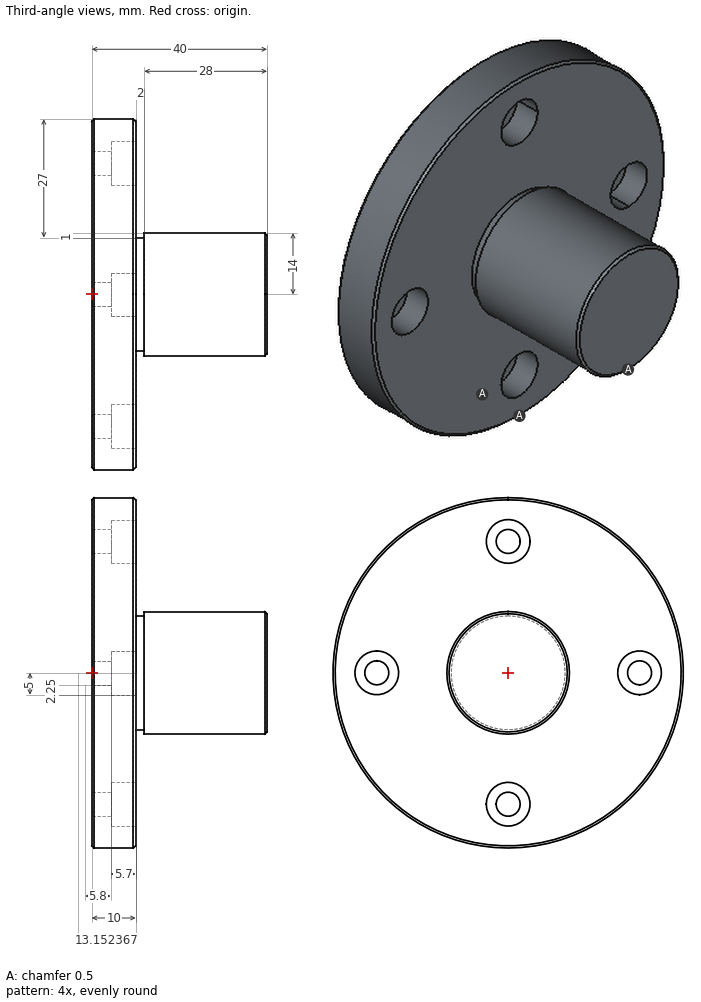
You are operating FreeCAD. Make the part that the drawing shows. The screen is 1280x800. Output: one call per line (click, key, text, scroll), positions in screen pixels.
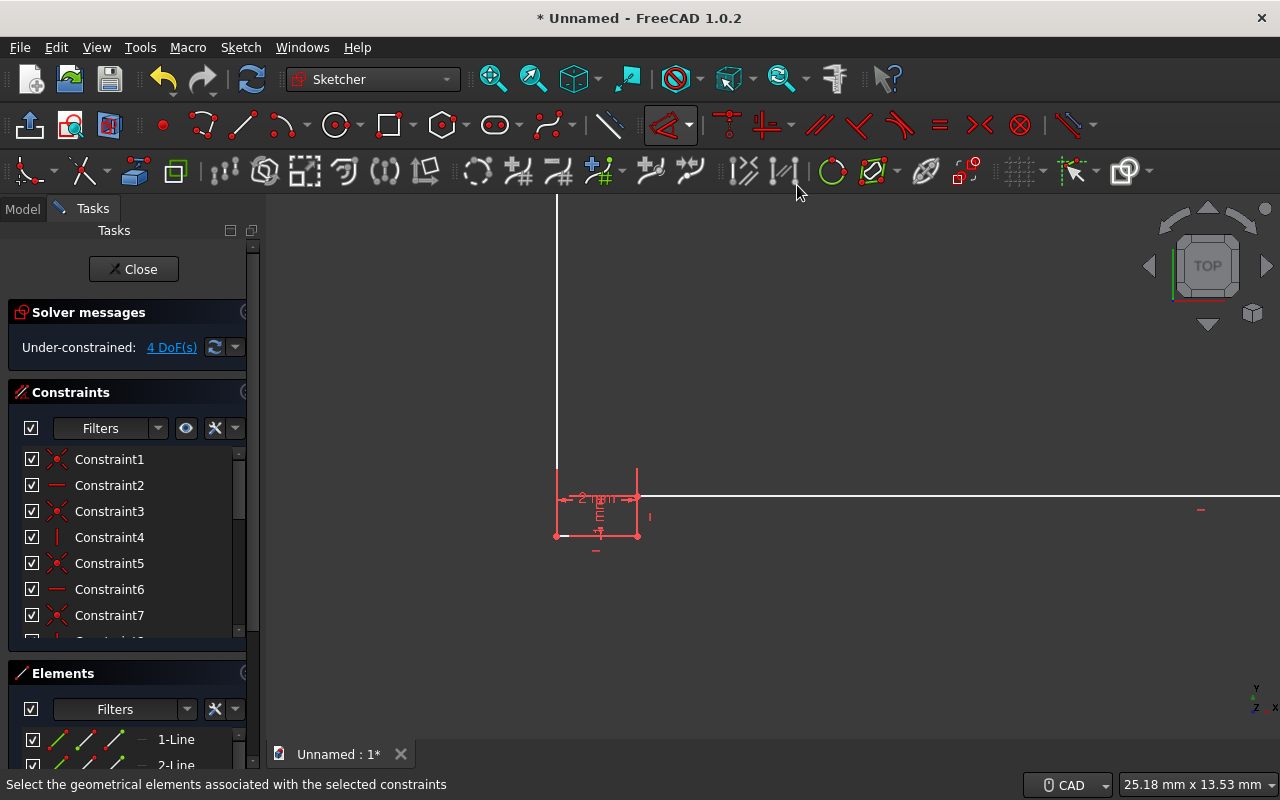
scroll(640, 520, down, 8)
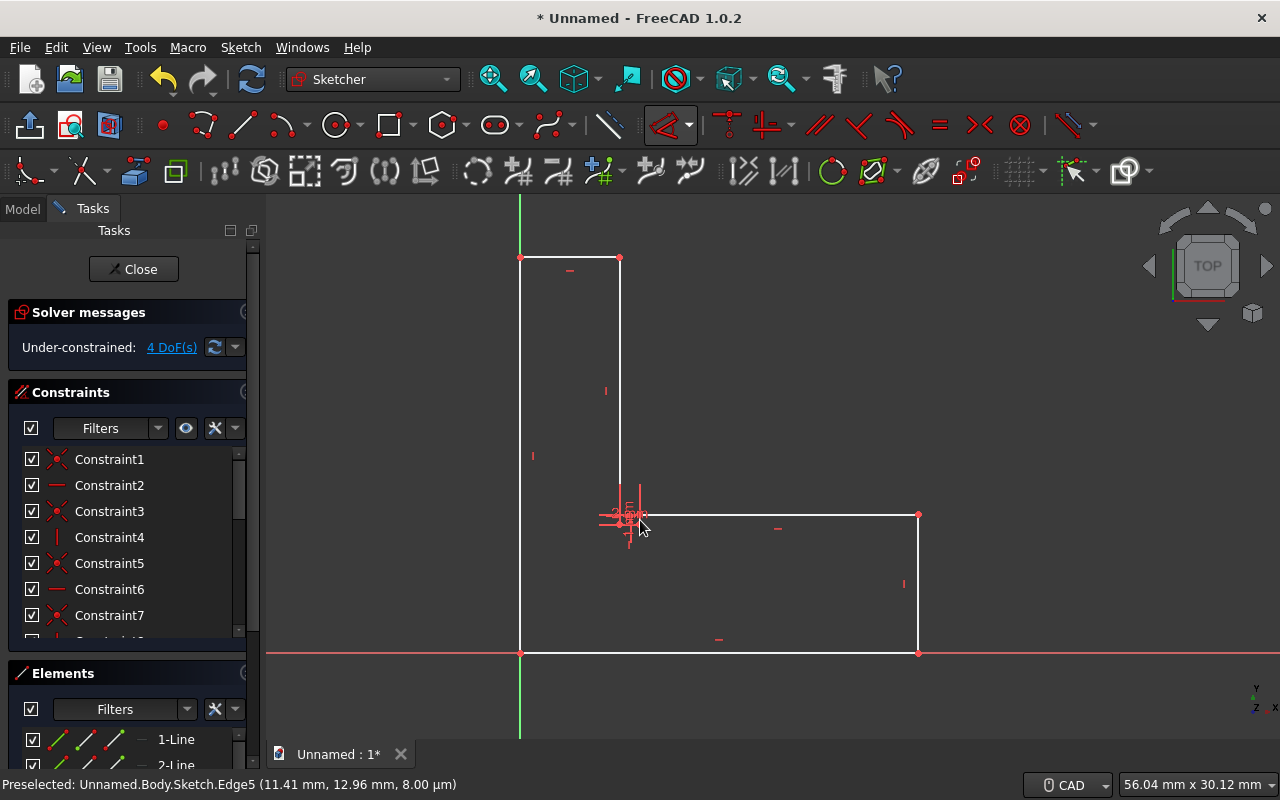
click(640, 629)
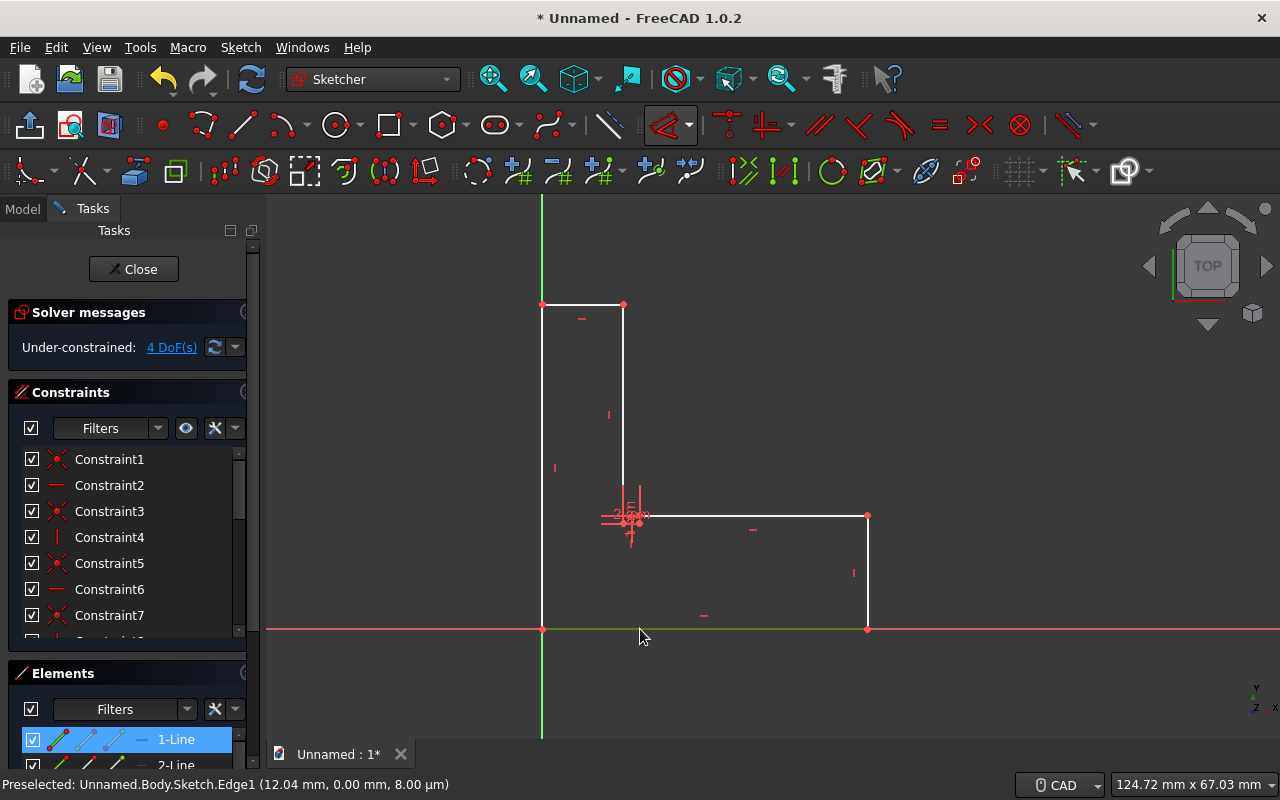
click(692, 126)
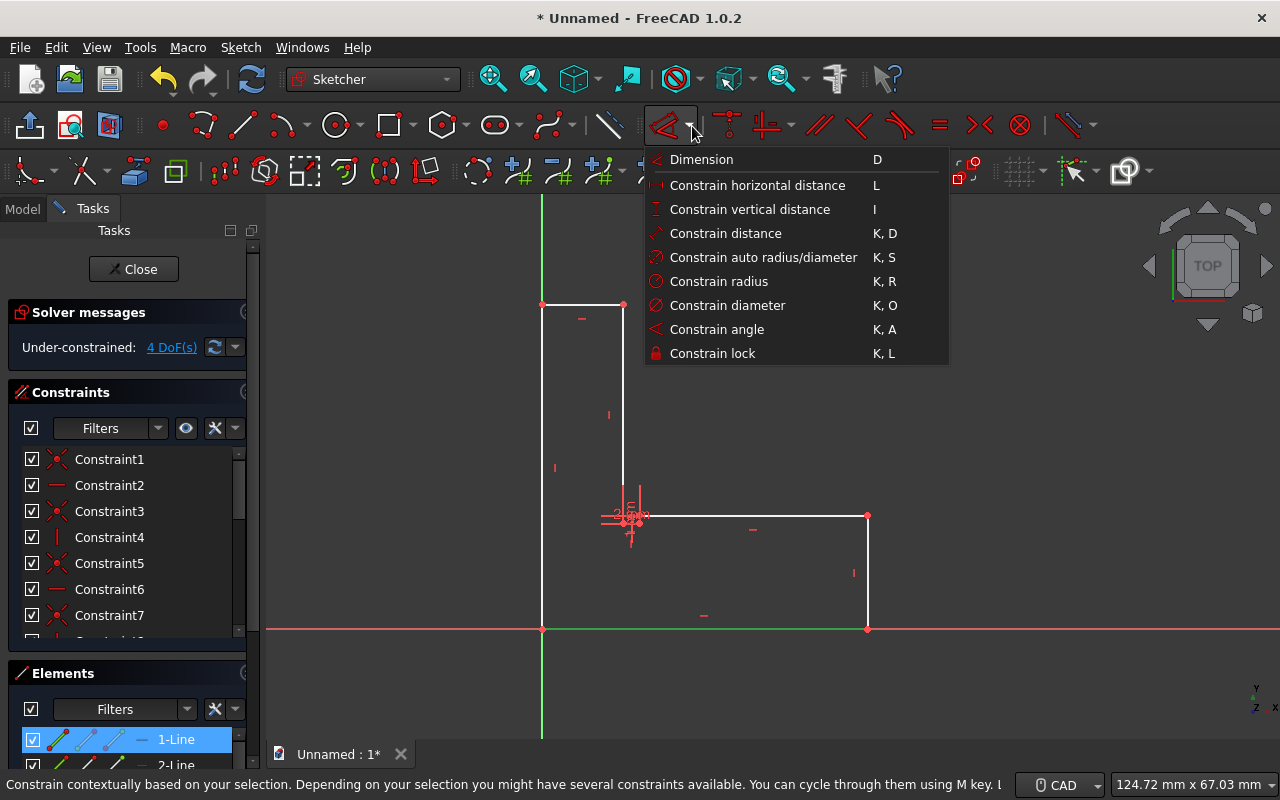
click(797, 185)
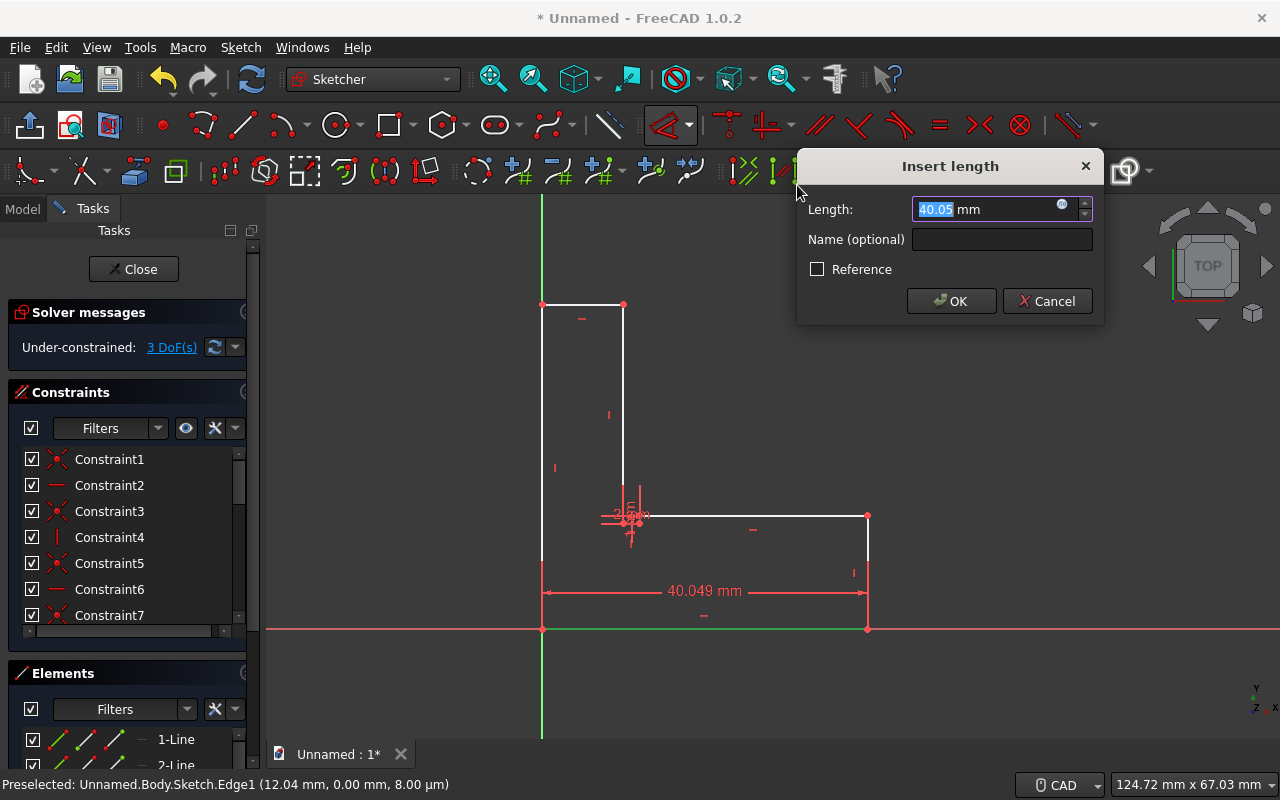
text(40)
key(Return)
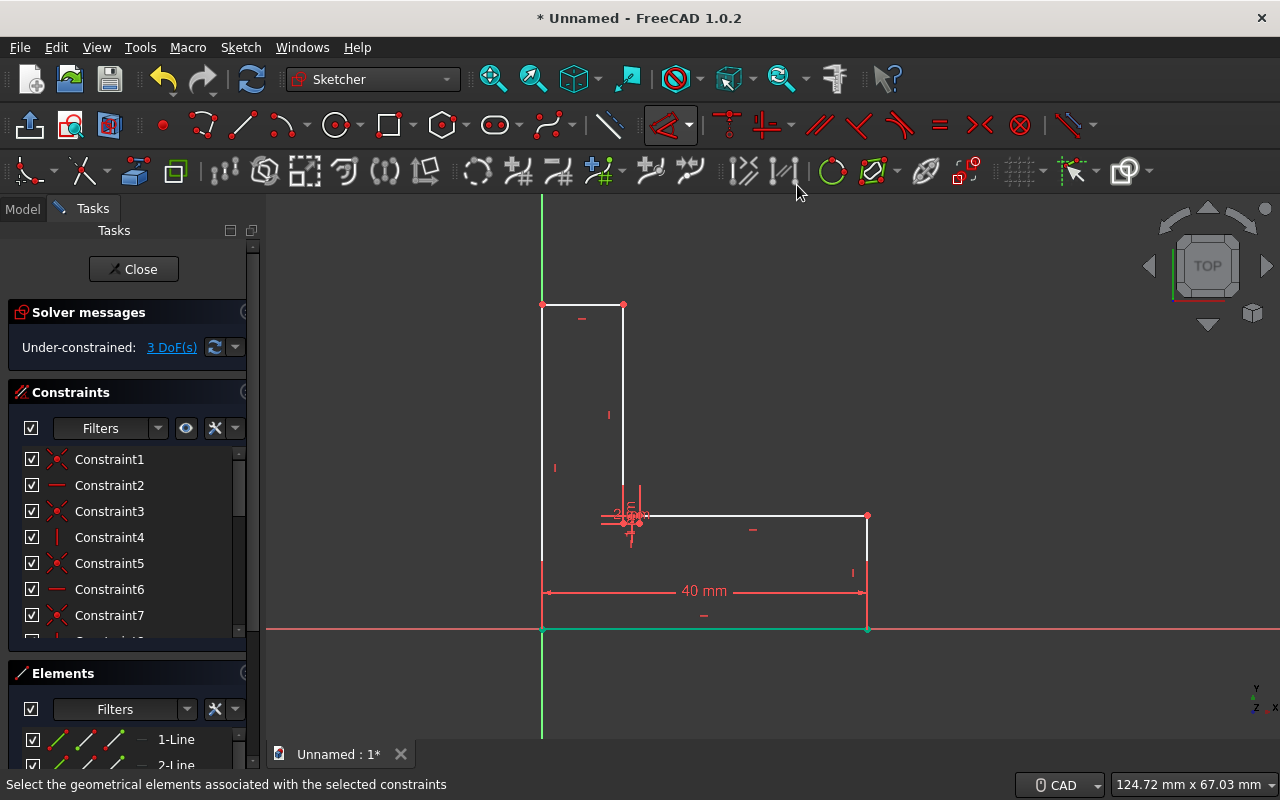
click(867, 595)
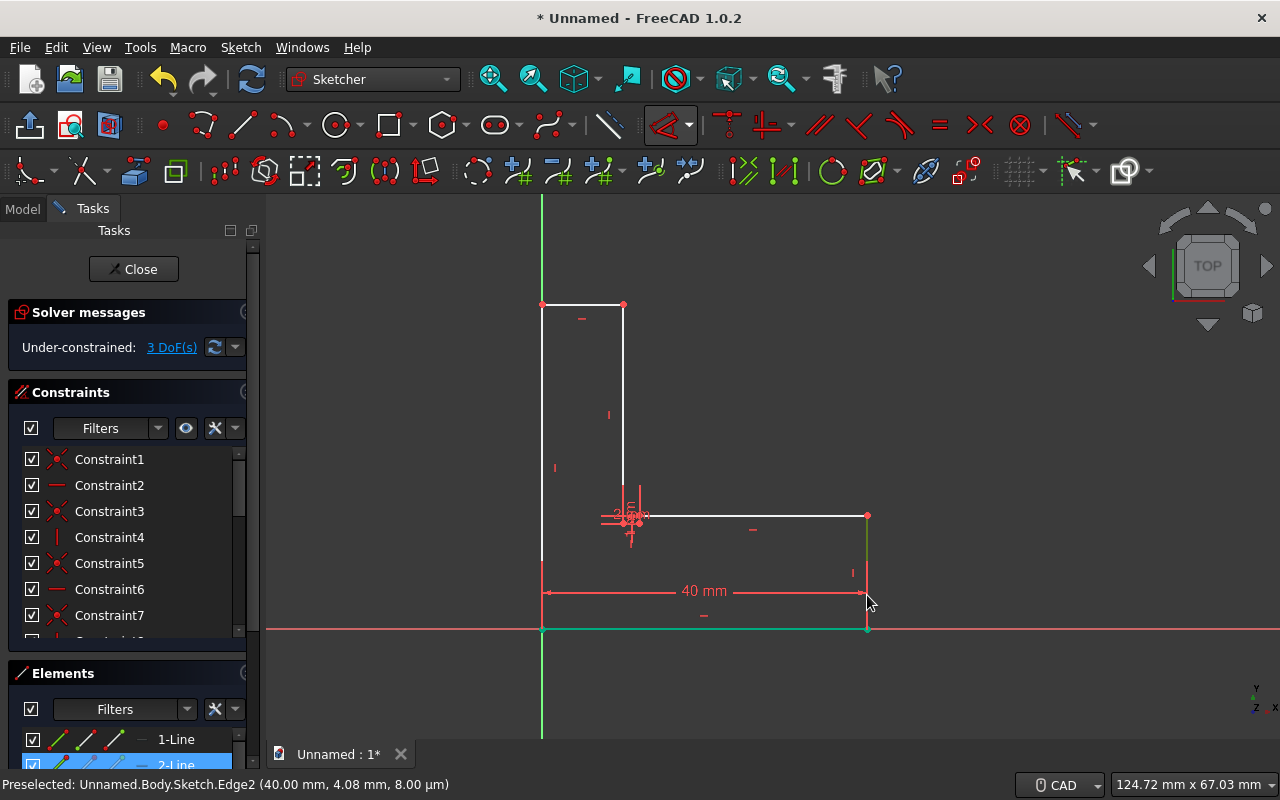
key(i)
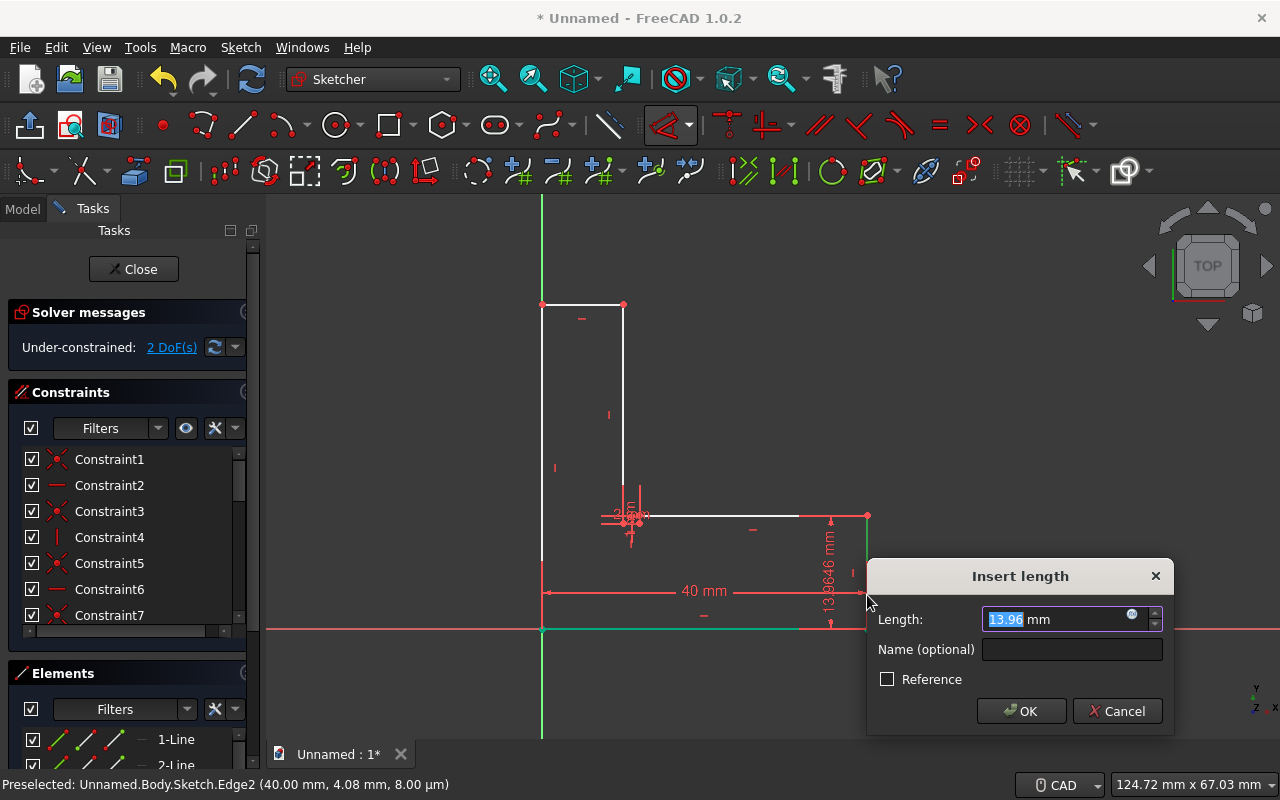
text(14)
key(Return)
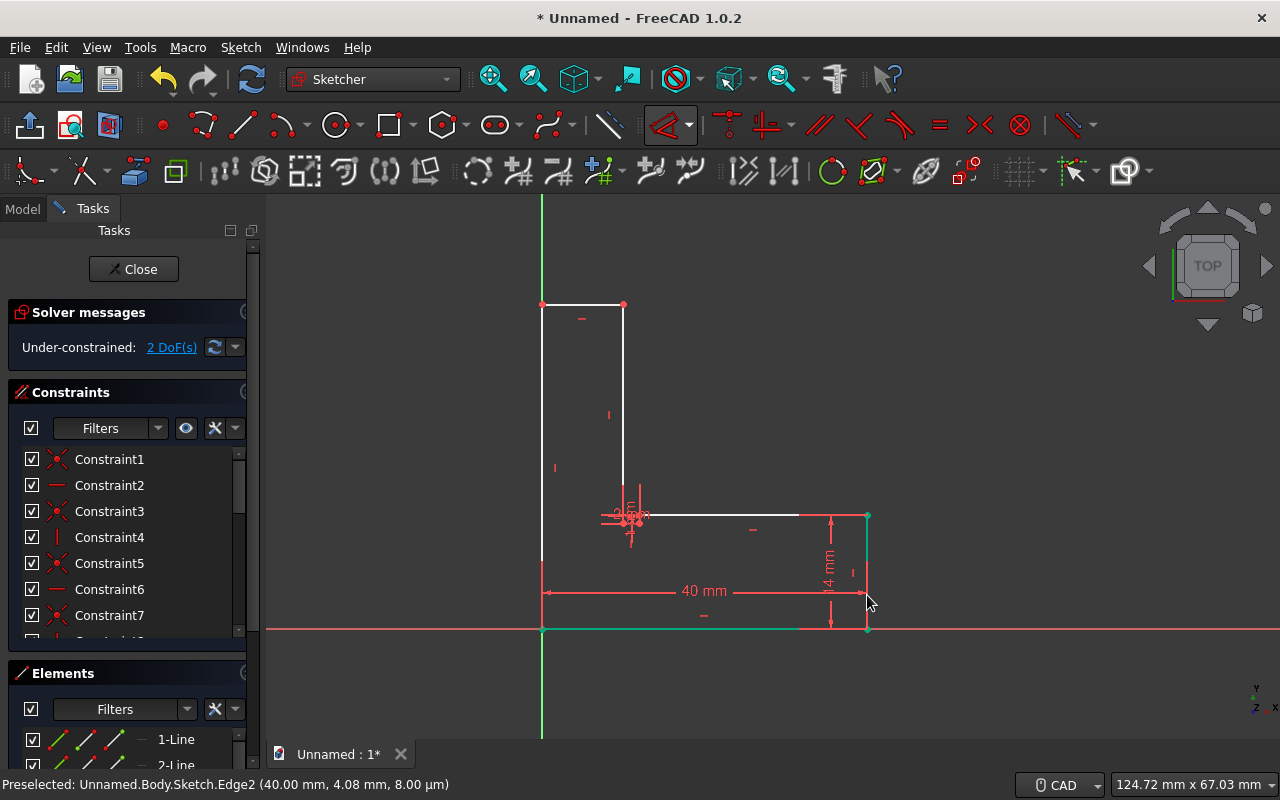
click(799, 515)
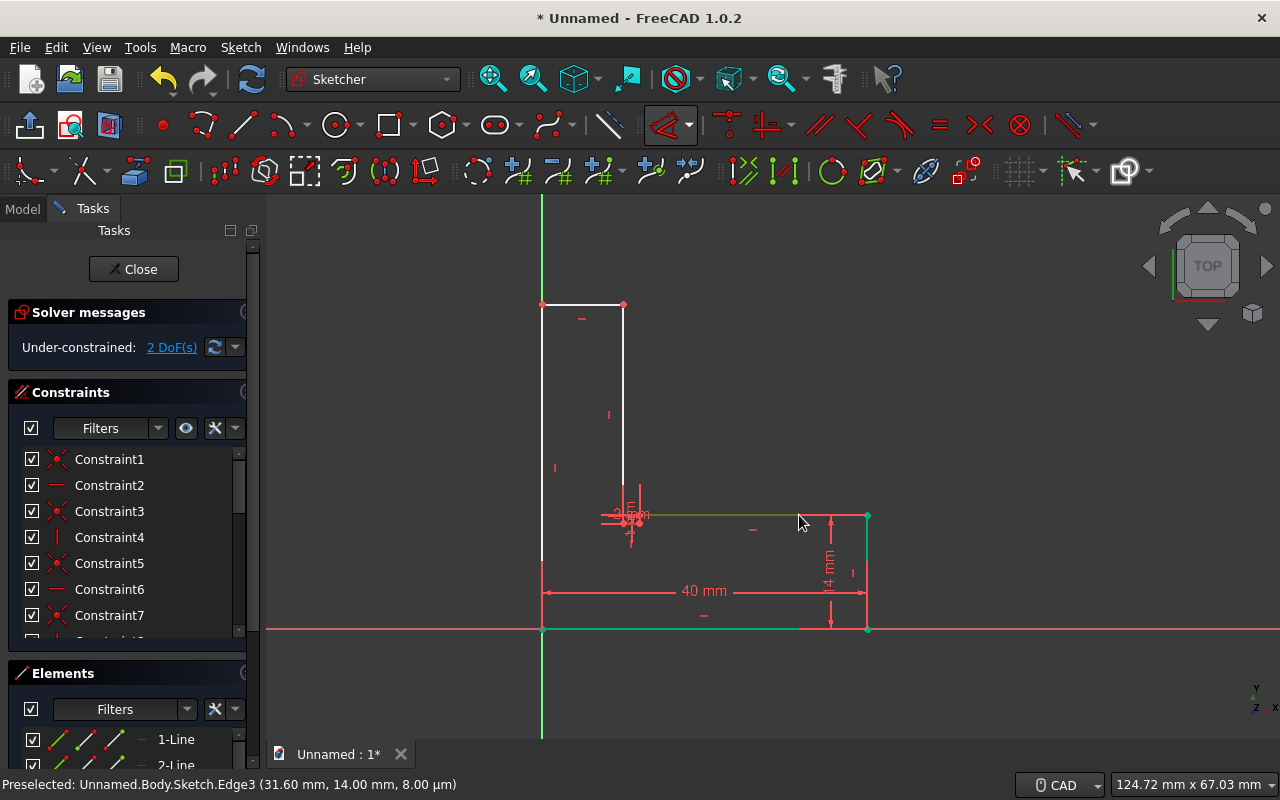
click(692, 126)